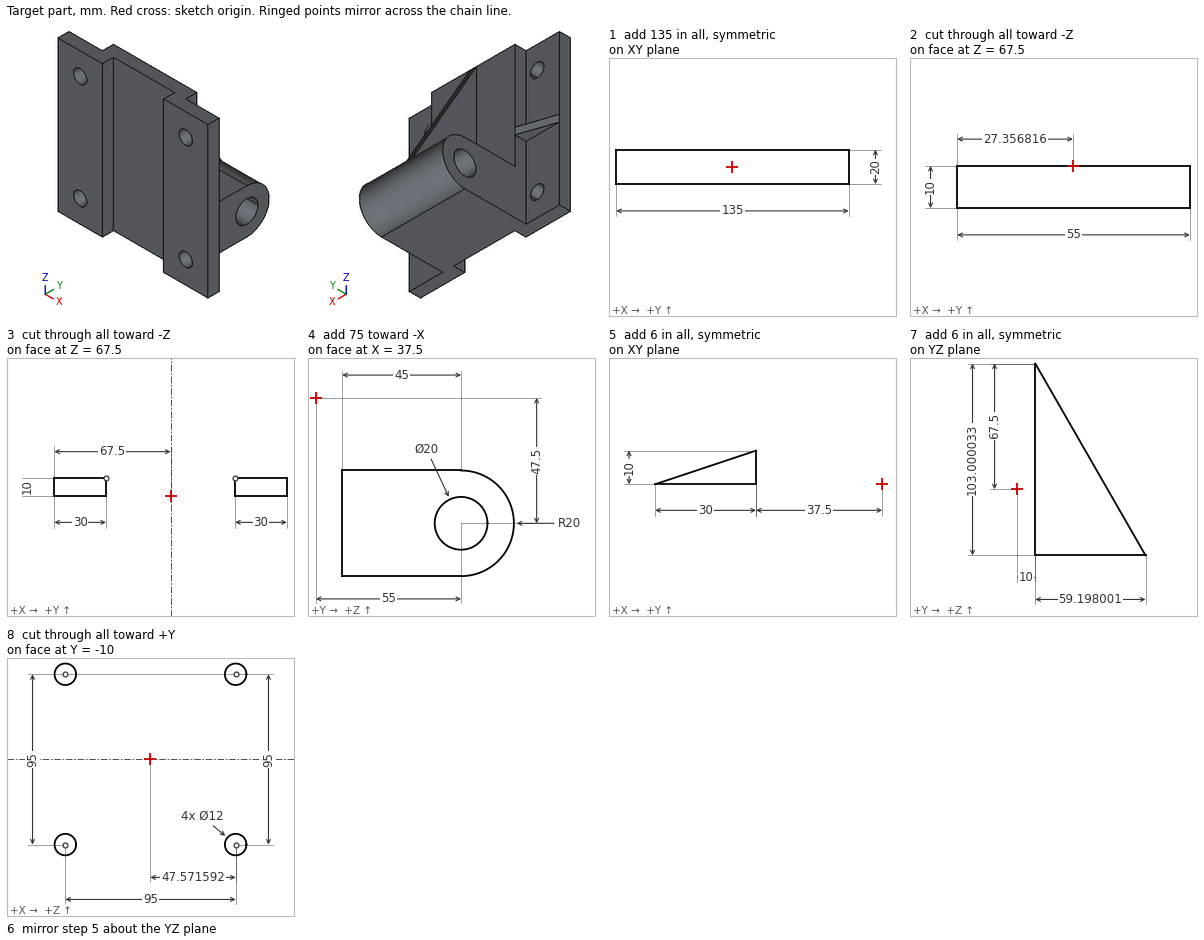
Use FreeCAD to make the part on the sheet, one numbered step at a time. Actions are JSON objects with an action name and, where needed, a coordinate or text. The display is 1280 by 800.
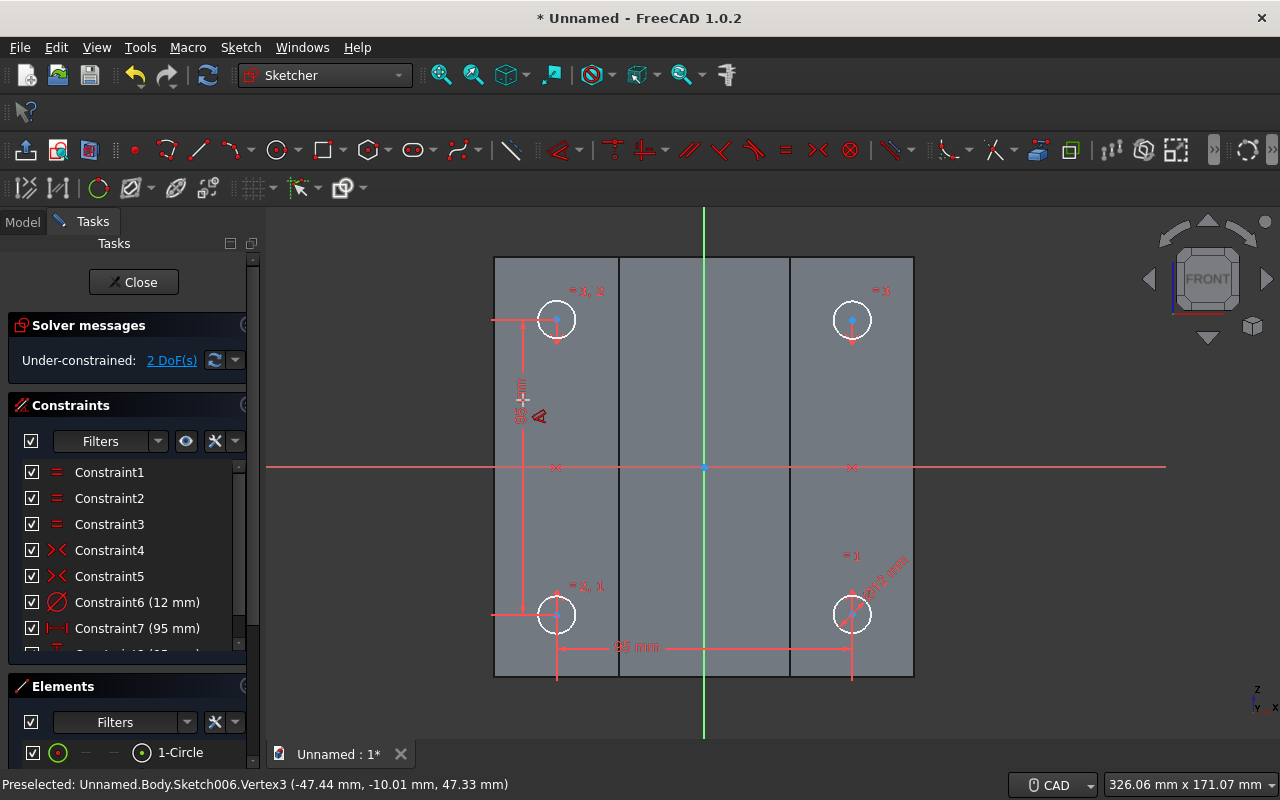
{"action": "left_click", "coordinate": [852, 614]}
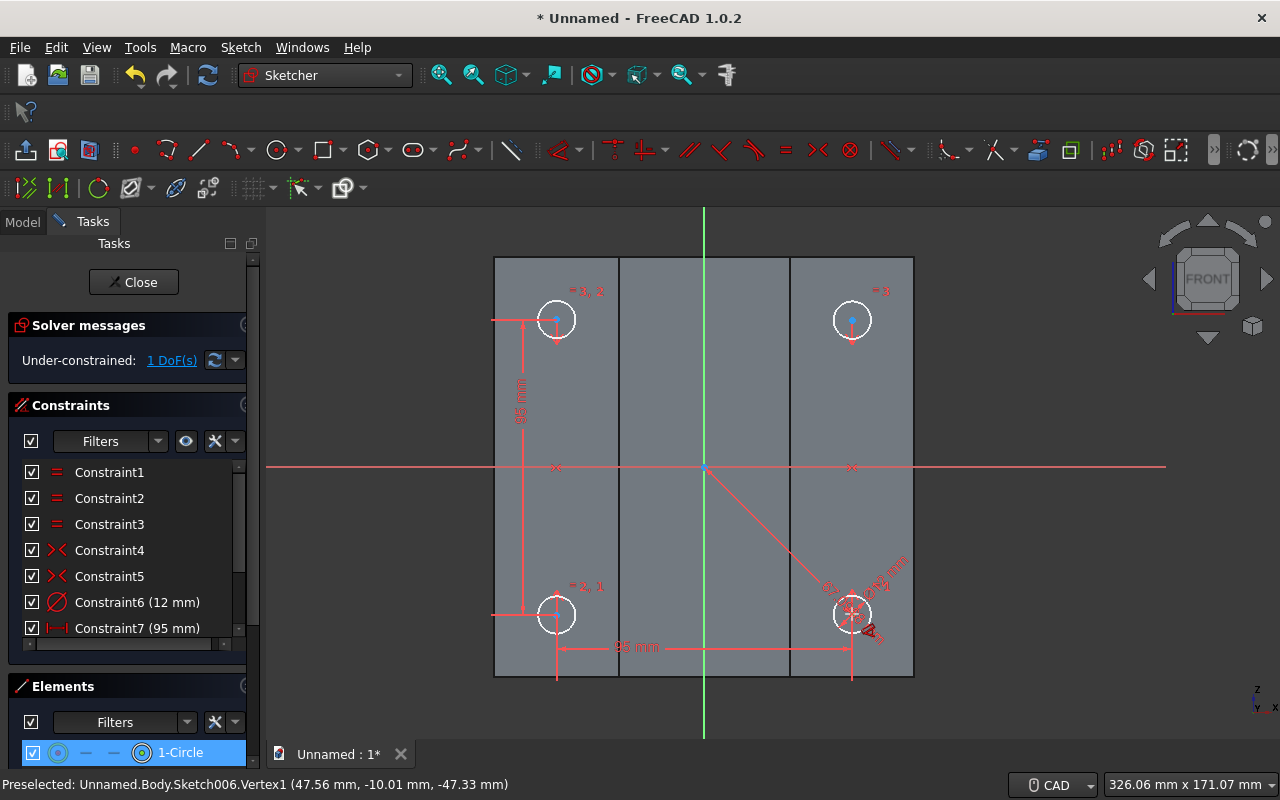
{"action": "left_click", "coordinate": [557, 320]}
{"action": "left_click", "coordinate": [523, 535]}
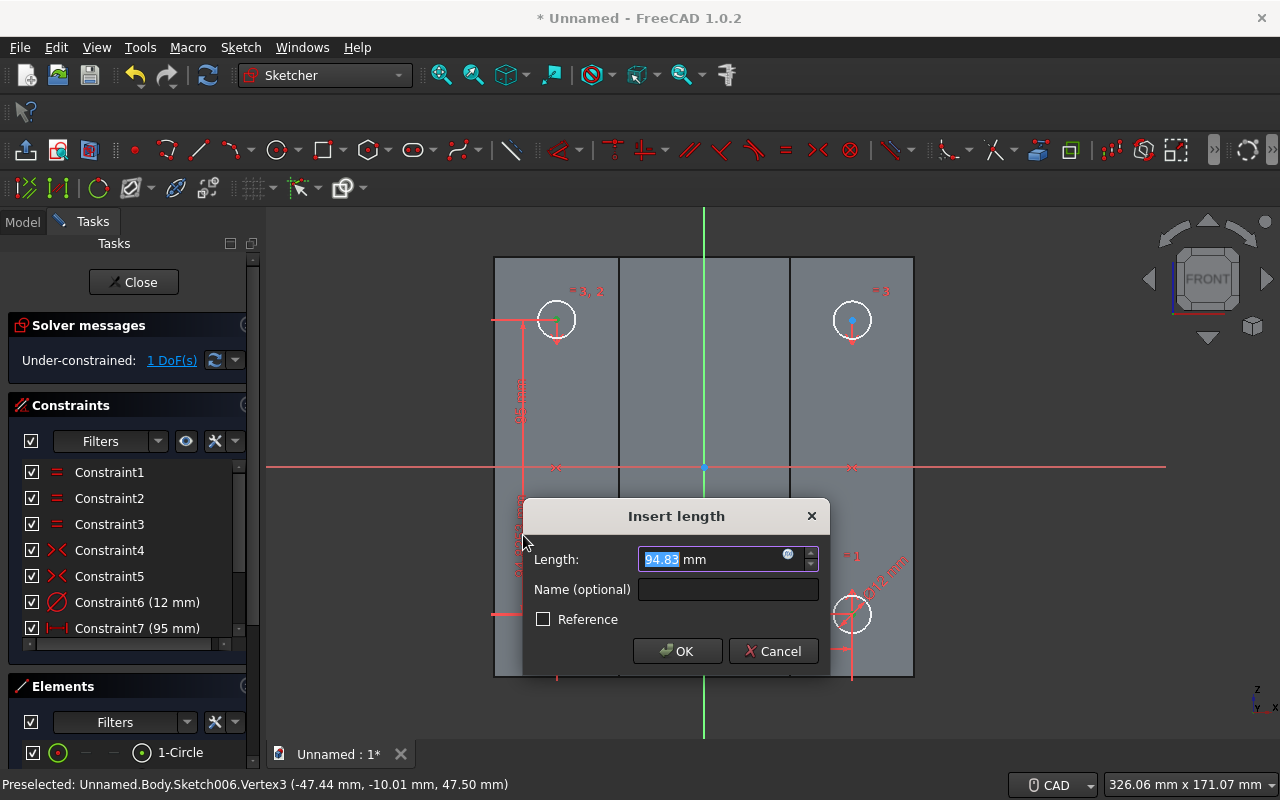
{"action": "type", "text": "95"}
{"action": "key", "text": "Return"}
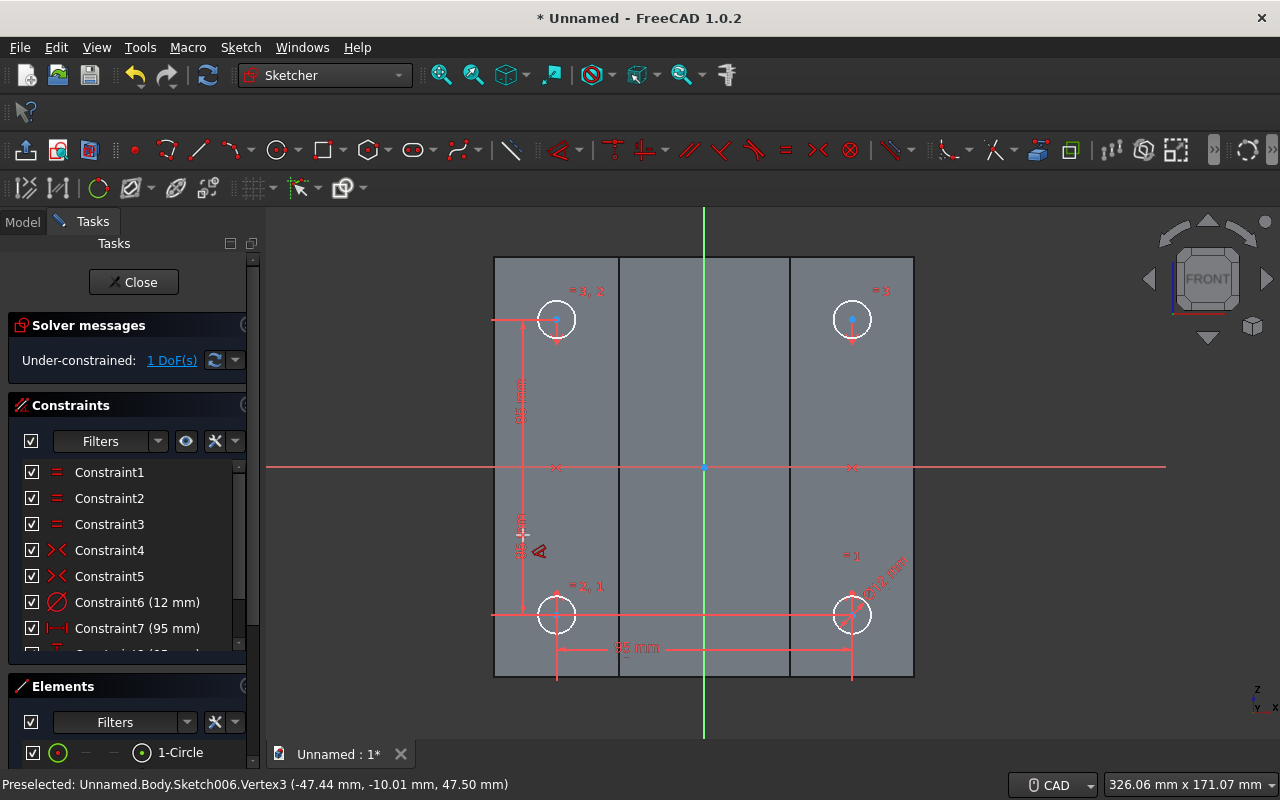
{"action": "left_click", "coordinate": [852, 615]}
{"action": "left_click", "coordinate": [778, 649]}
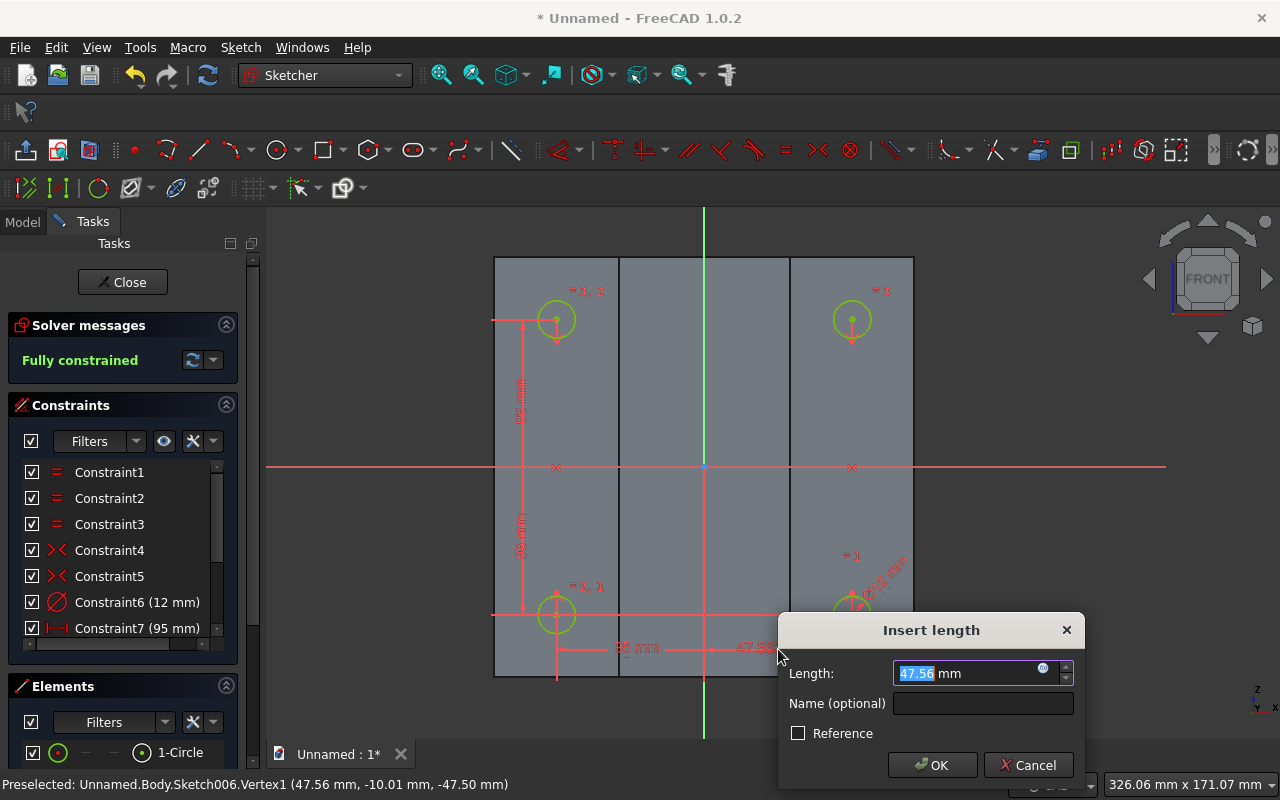
{"action": "type", "text": "47.571592"}
{"action": "key", "text": "Return"}
{"action": "key", "text": "Escape"}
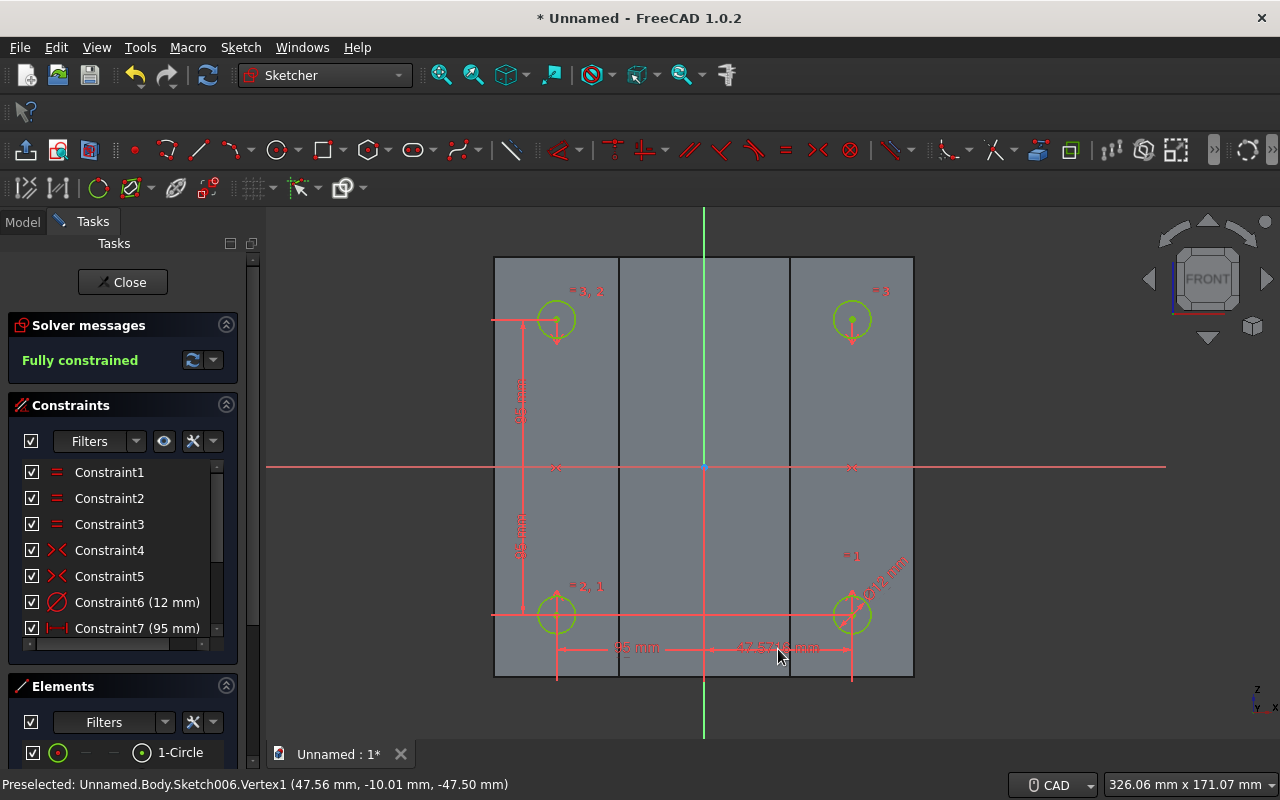
{"action": "left_click", "coordinate": [123, 282]}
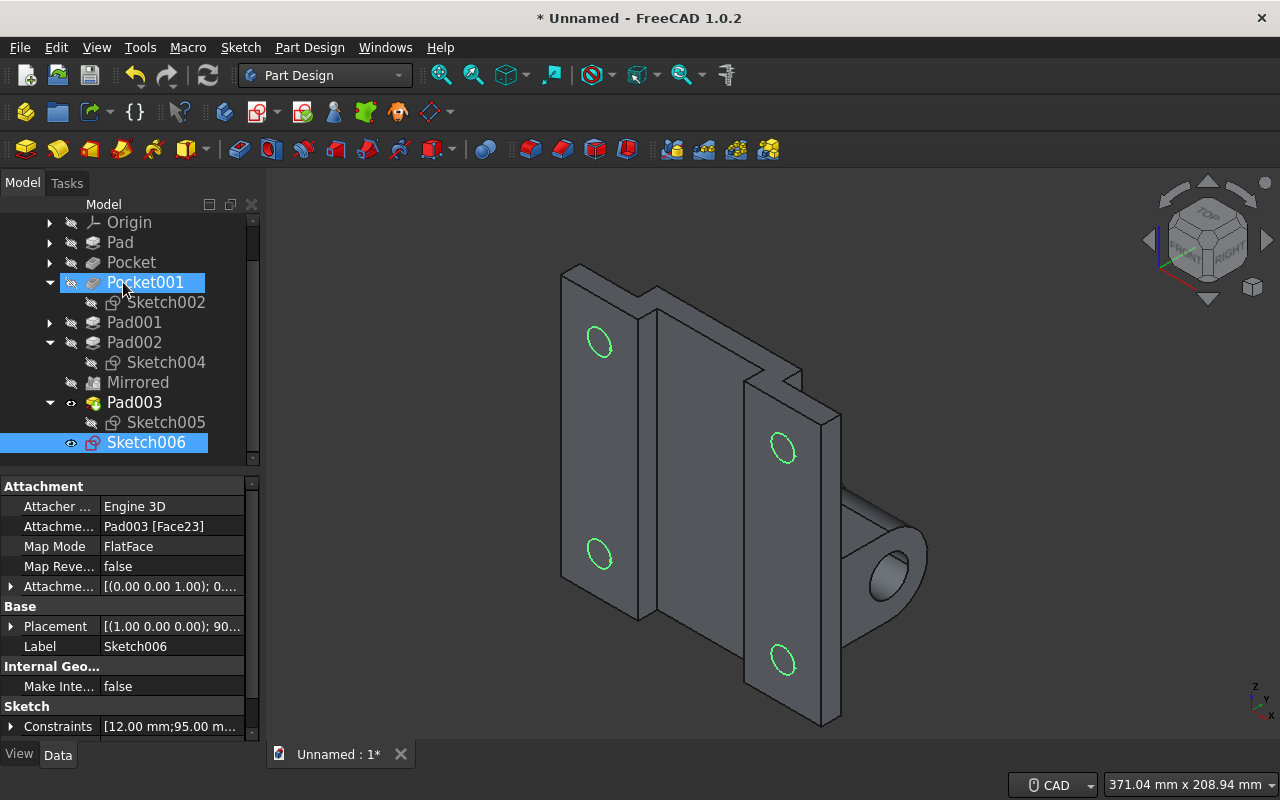
{"action": "left_click", "coordinate": [240, 150]}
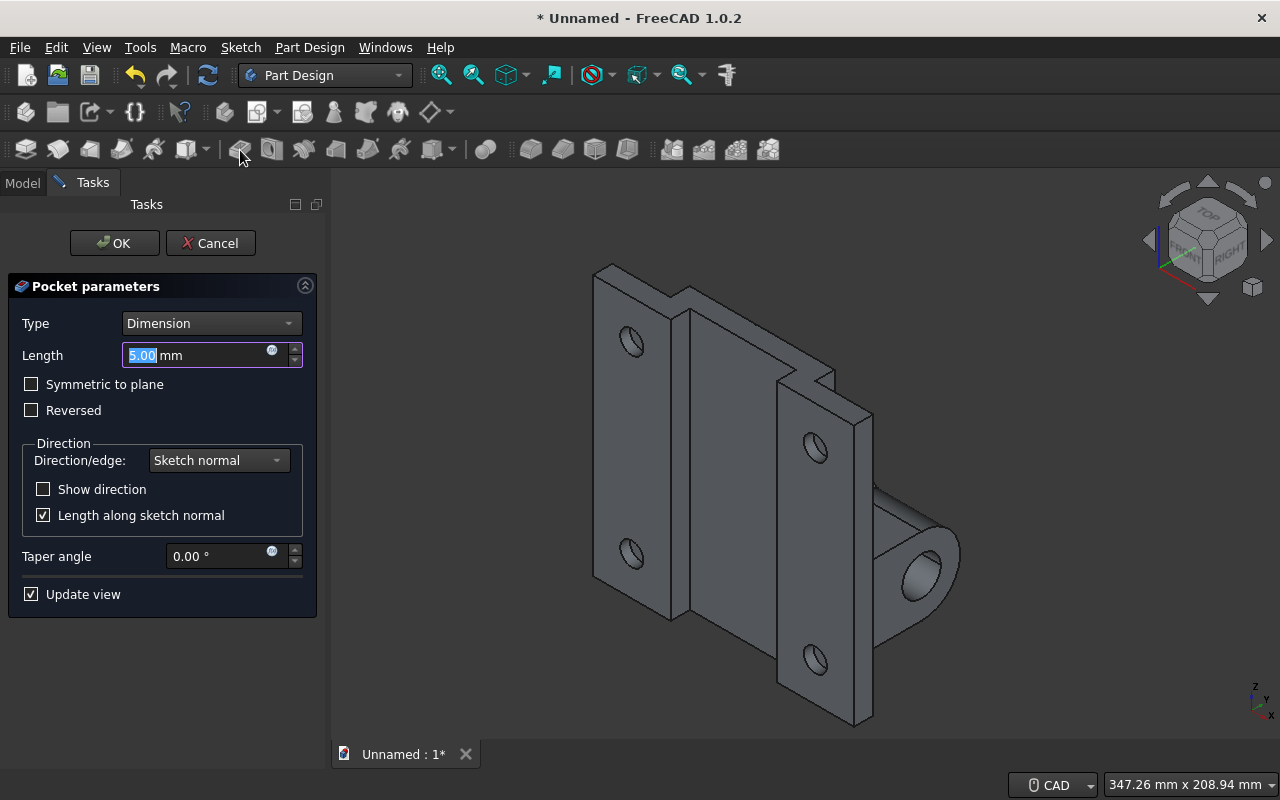
{"action": "left_click", "coordinate": [212, 324]}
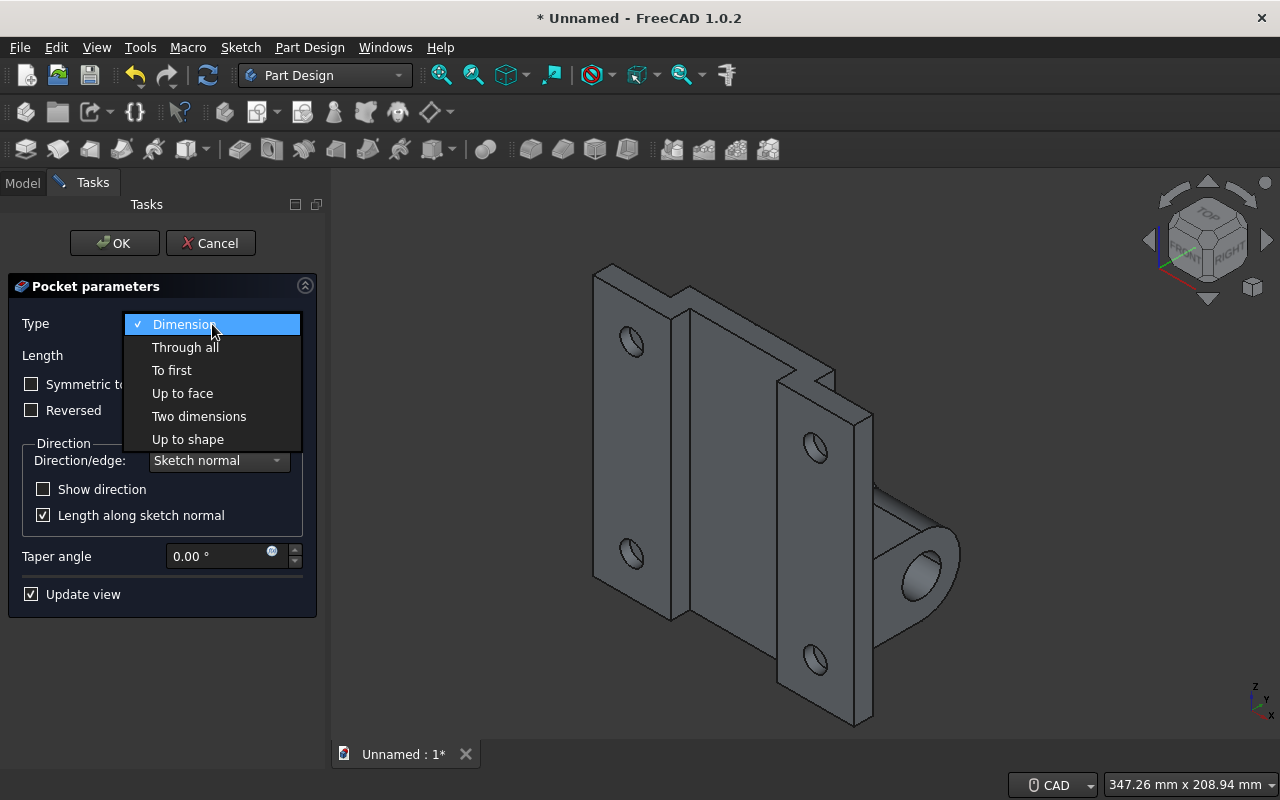
{"action": "left_click", "coordinate": [212, 348]}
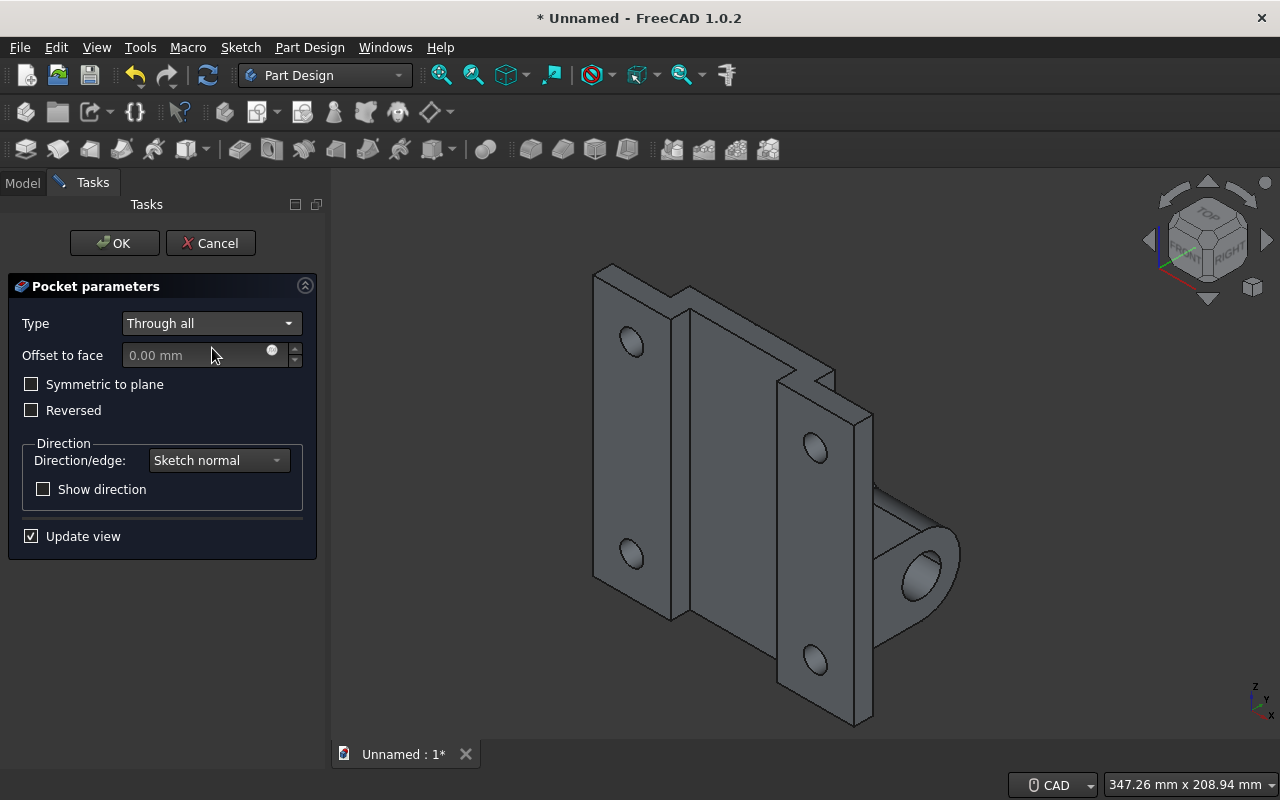
{"action": "left_click", "coordinate": [115, 243]}